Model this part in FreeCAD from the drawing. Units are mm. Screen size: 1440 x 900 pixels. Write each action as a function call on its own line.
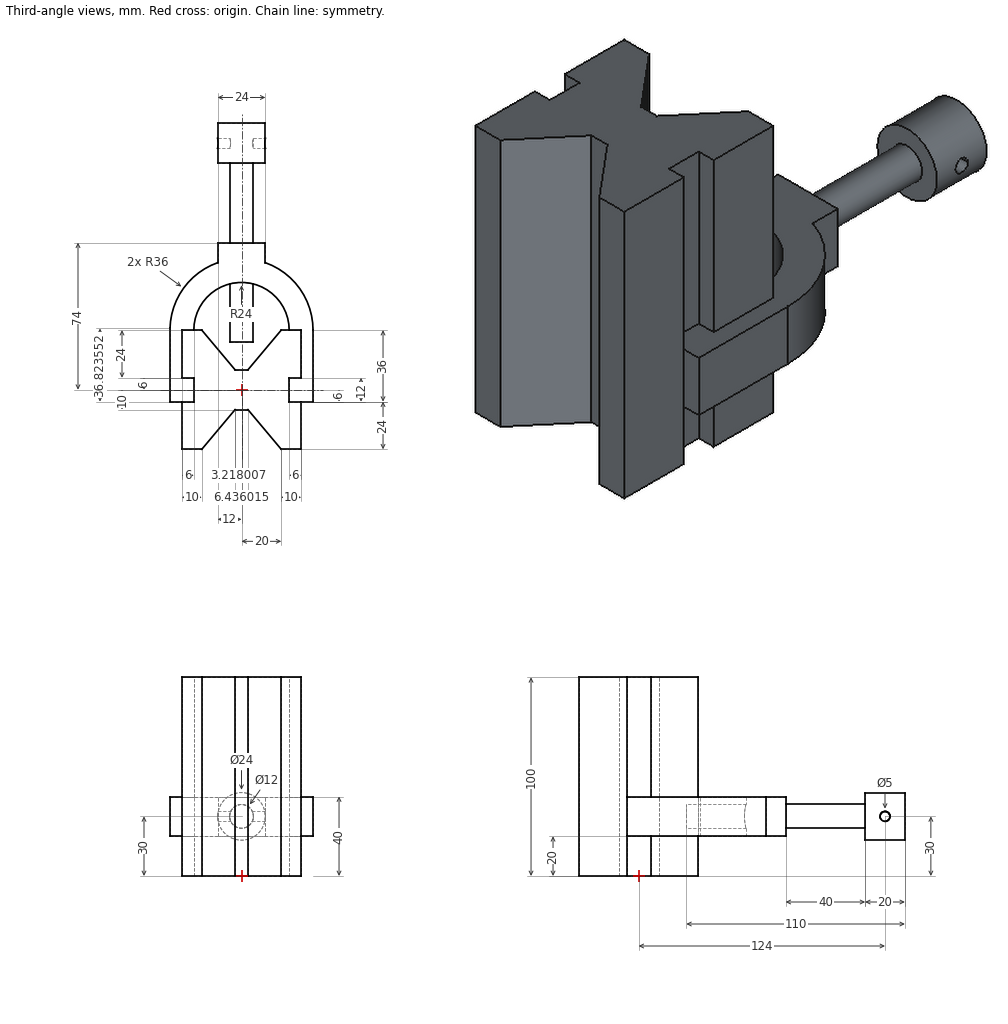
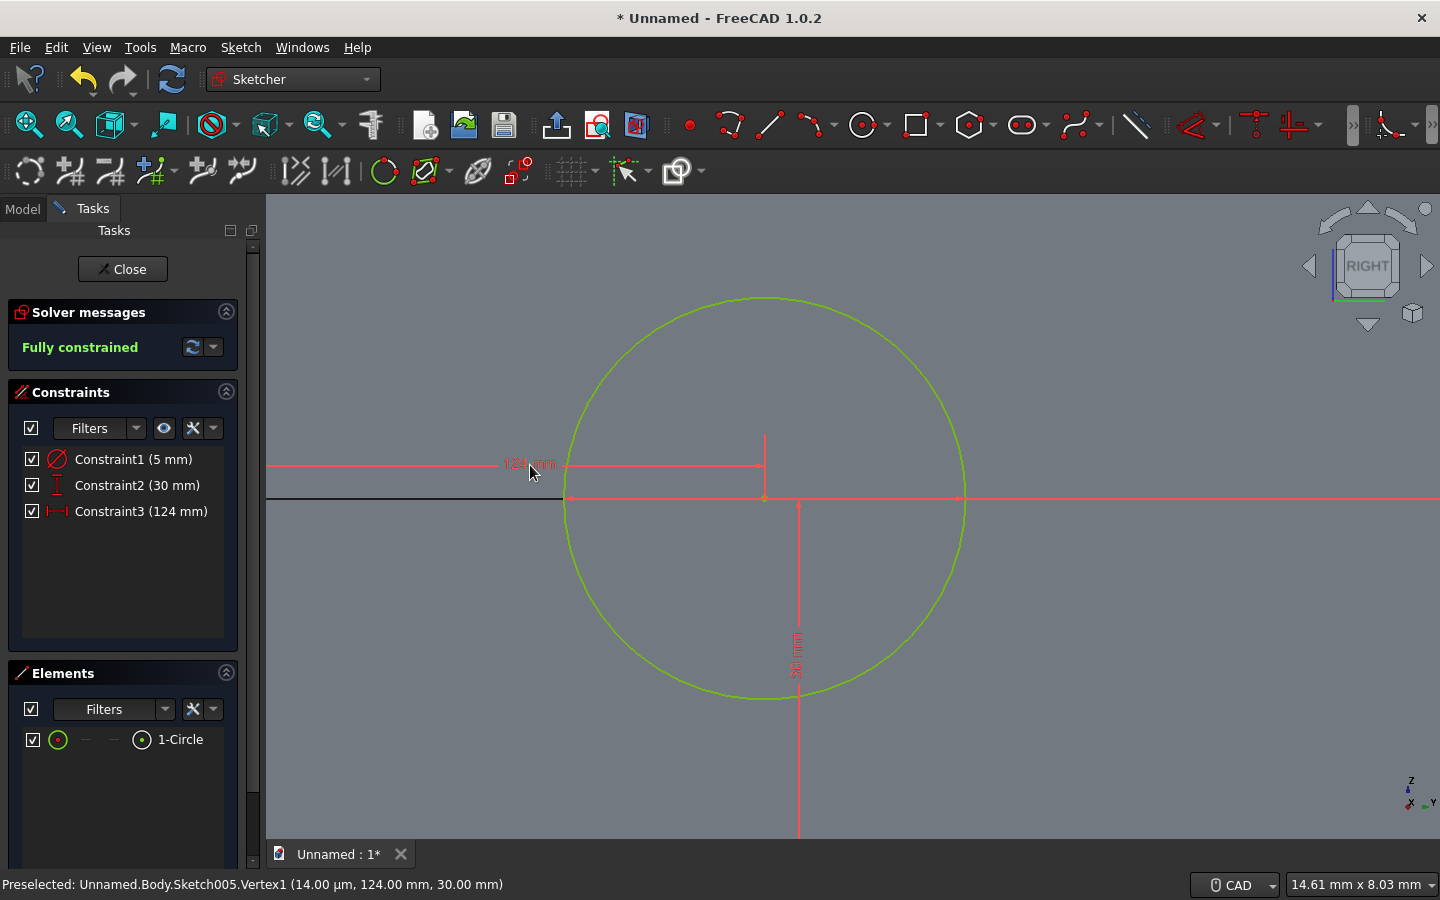
click(123, 269)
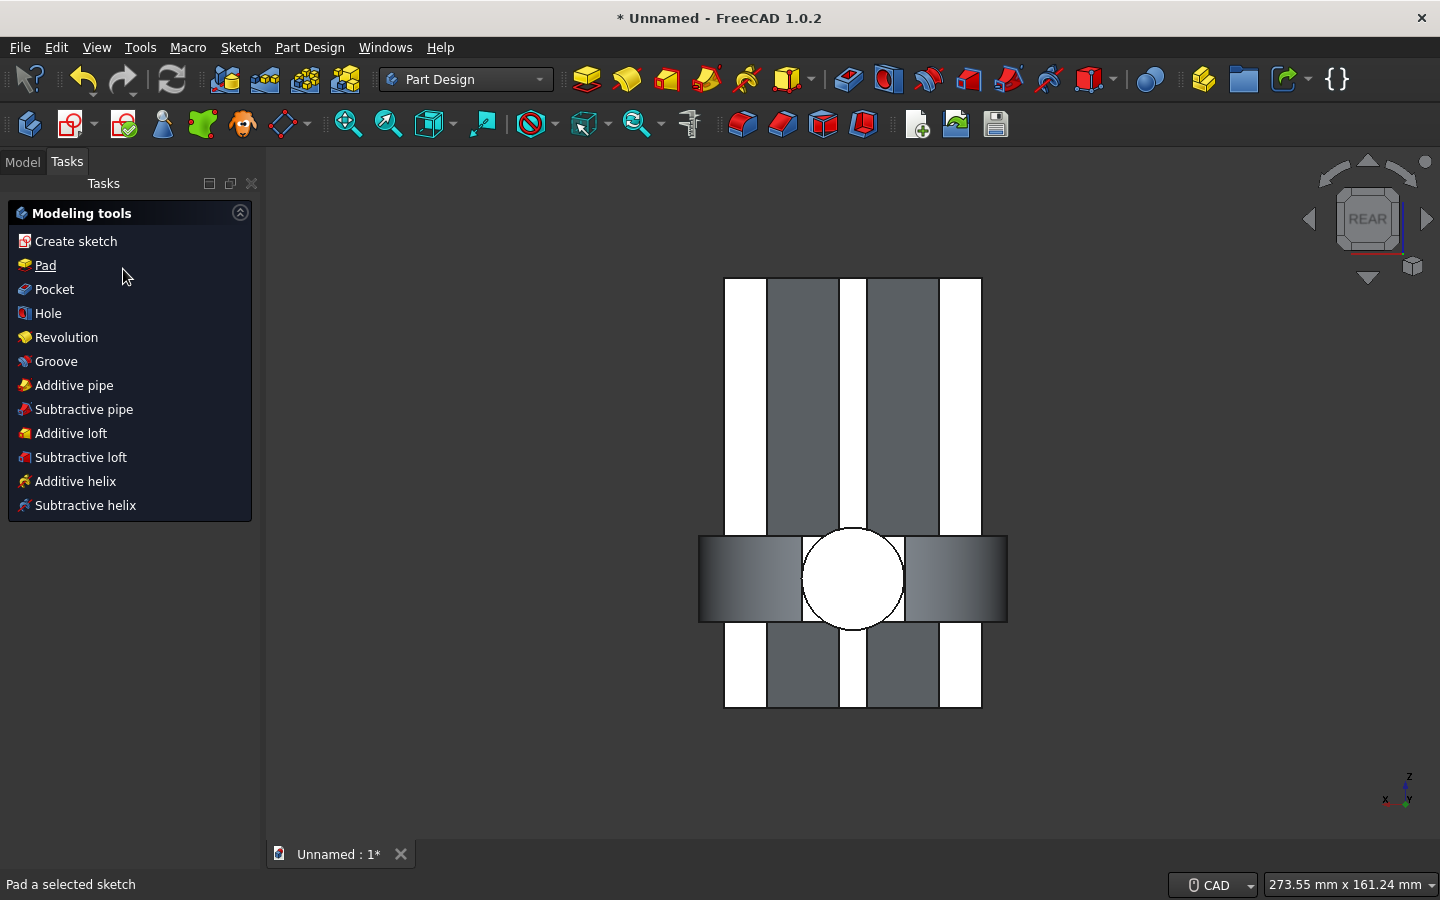
click(850, 80)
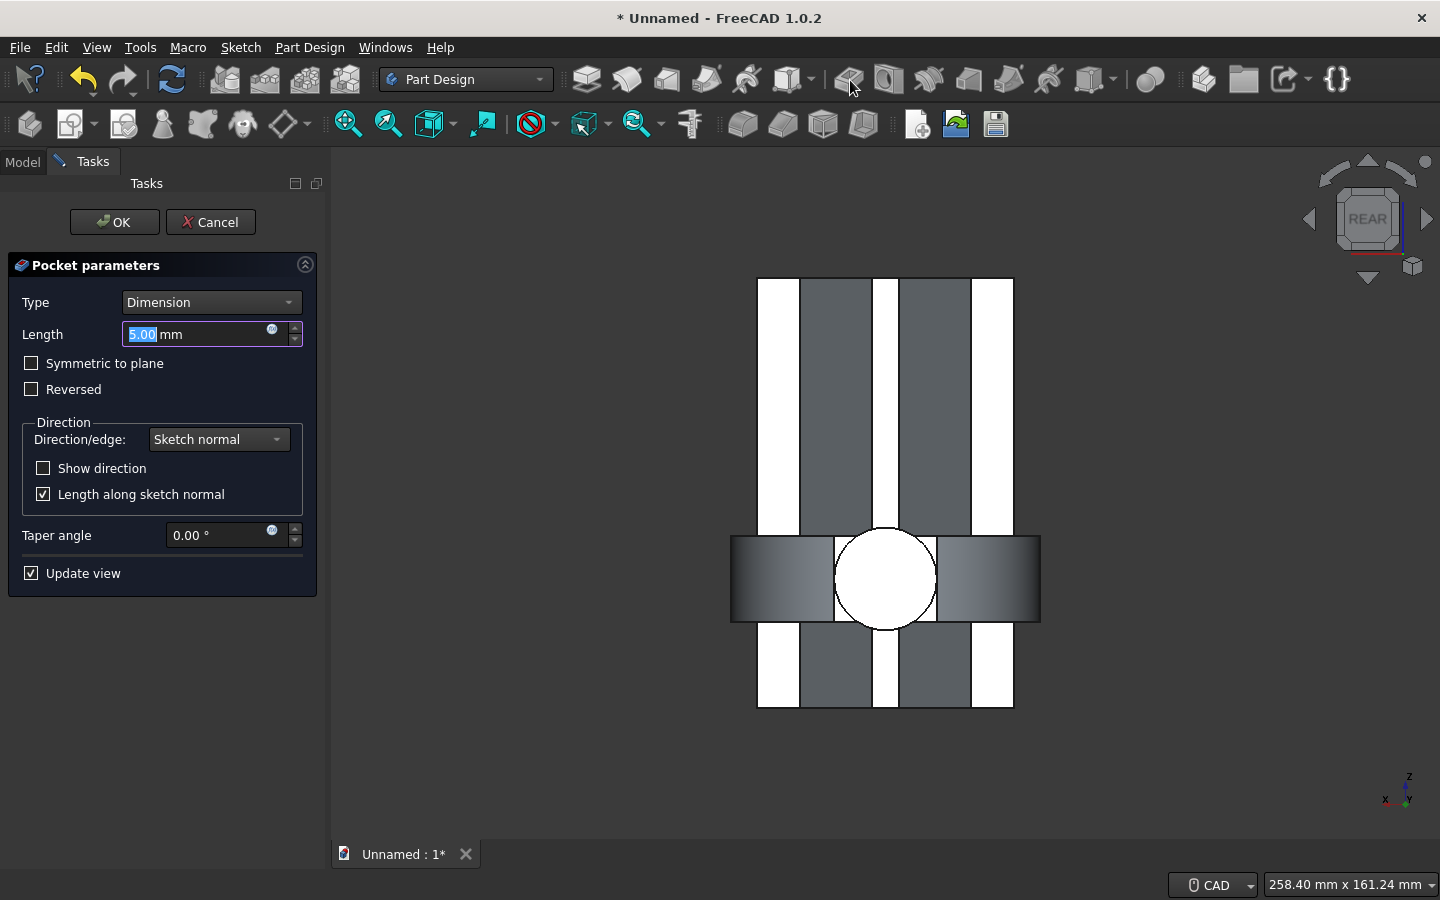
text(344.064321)
key(Tab)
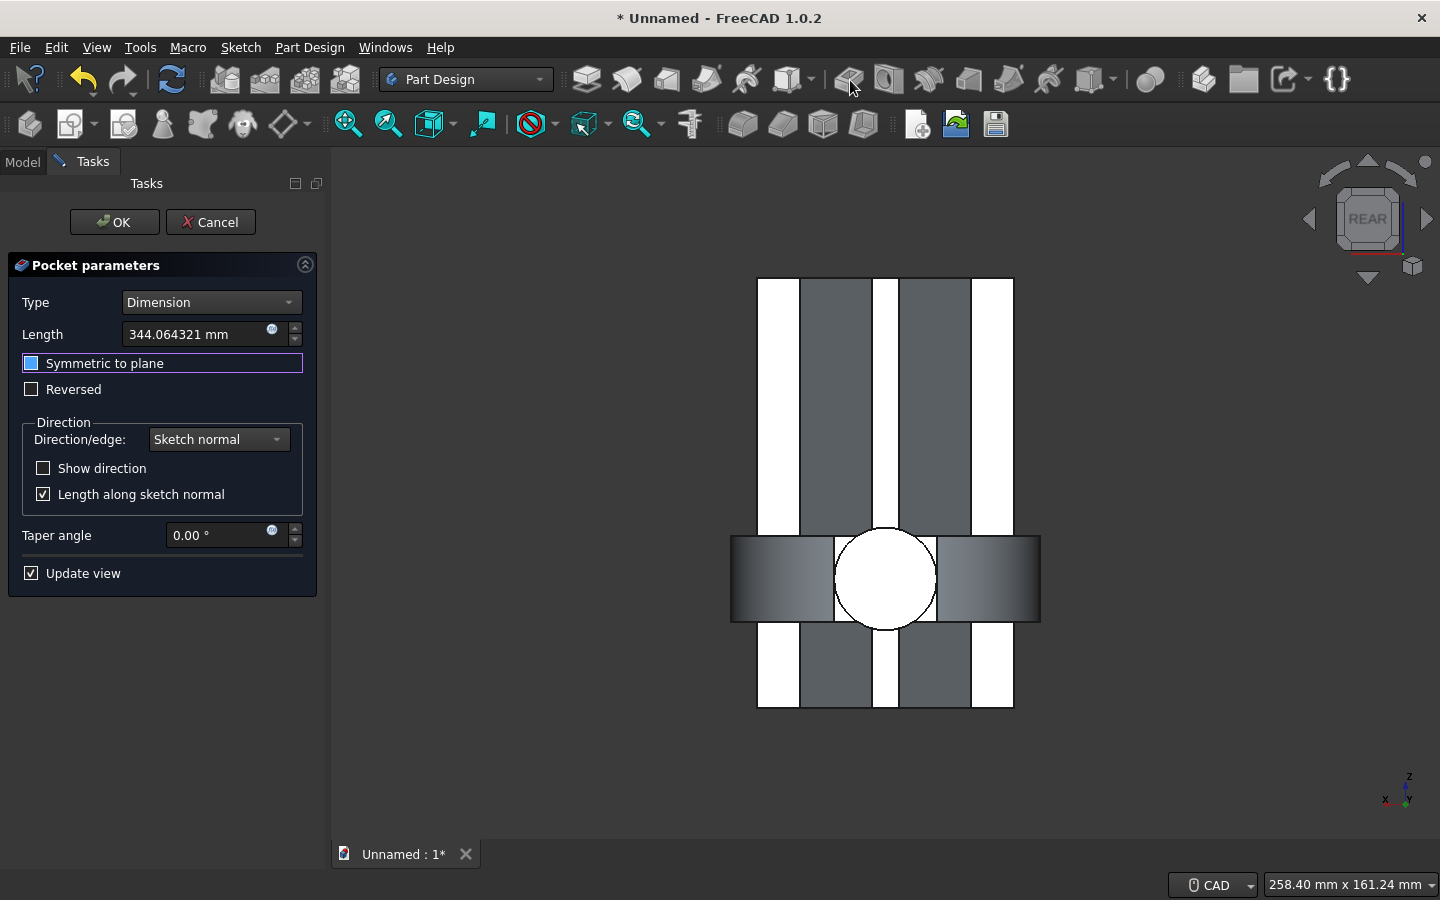
click(30, 363)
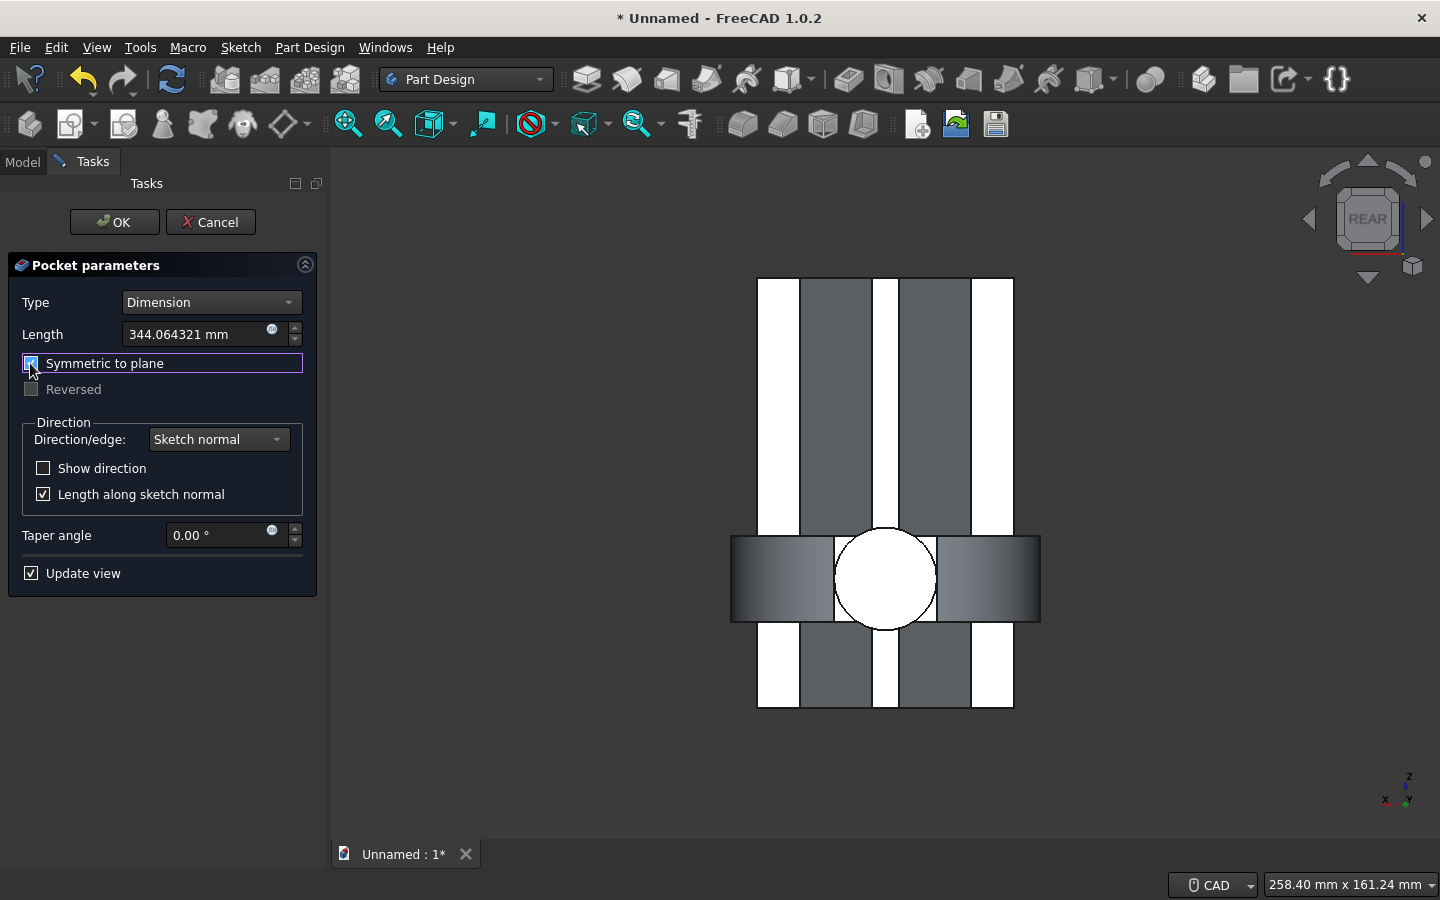
click(115, 222)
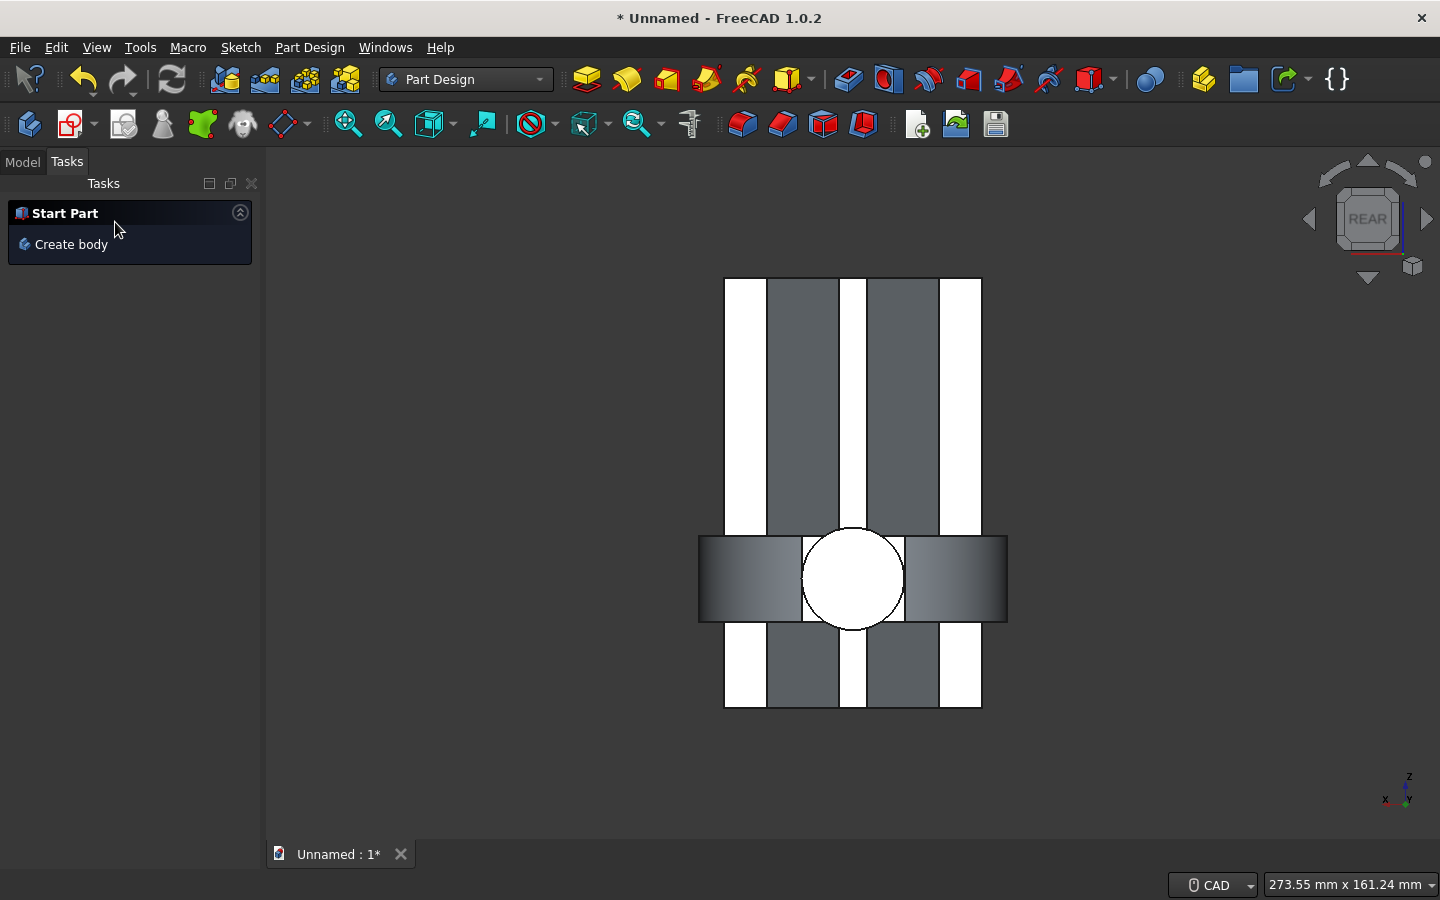
click(23, 161)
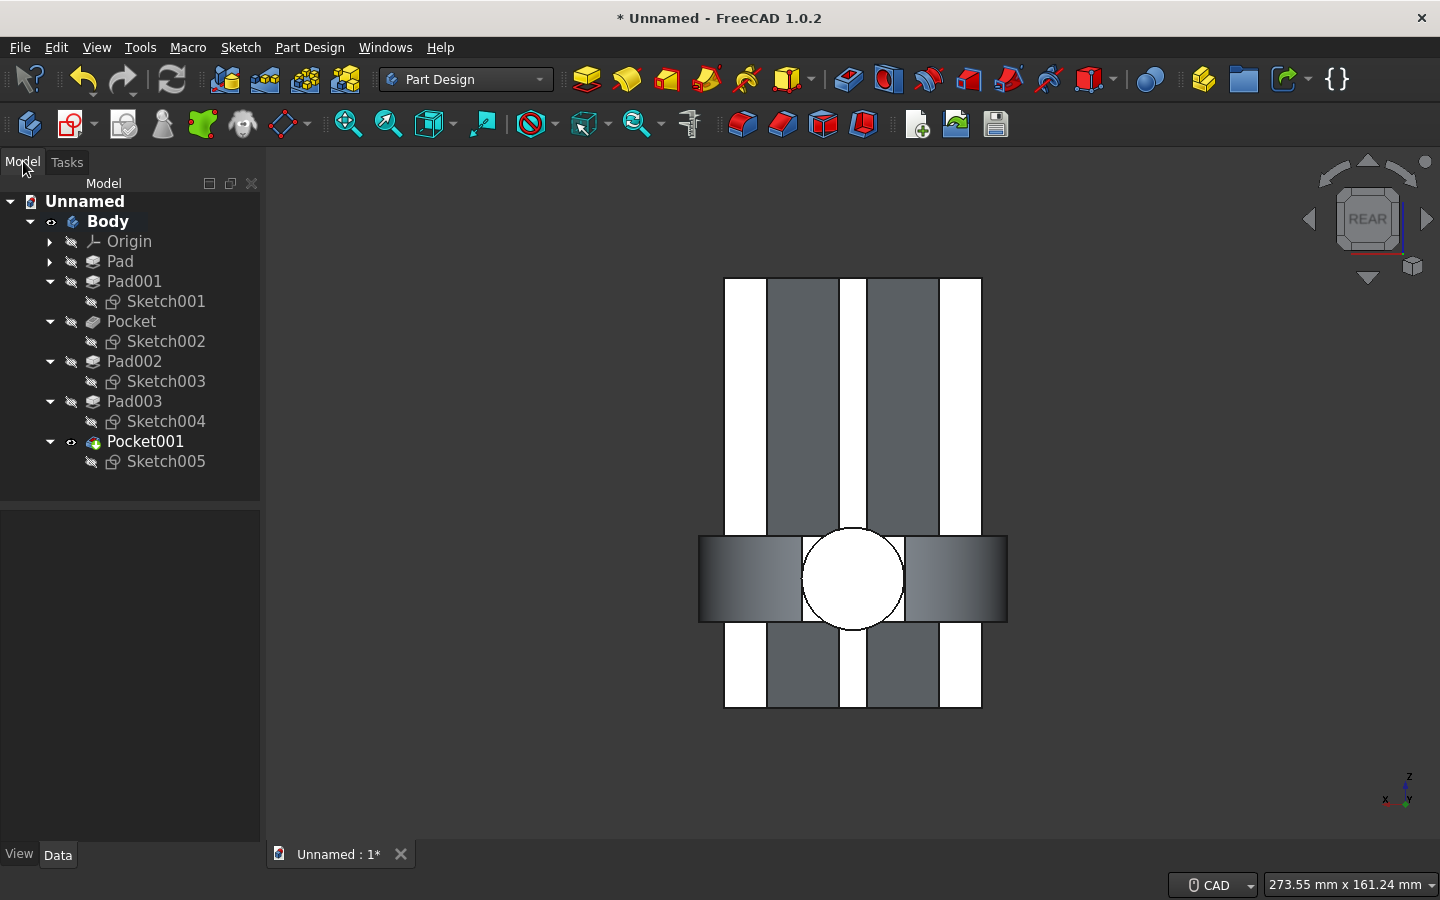
click(50, 242)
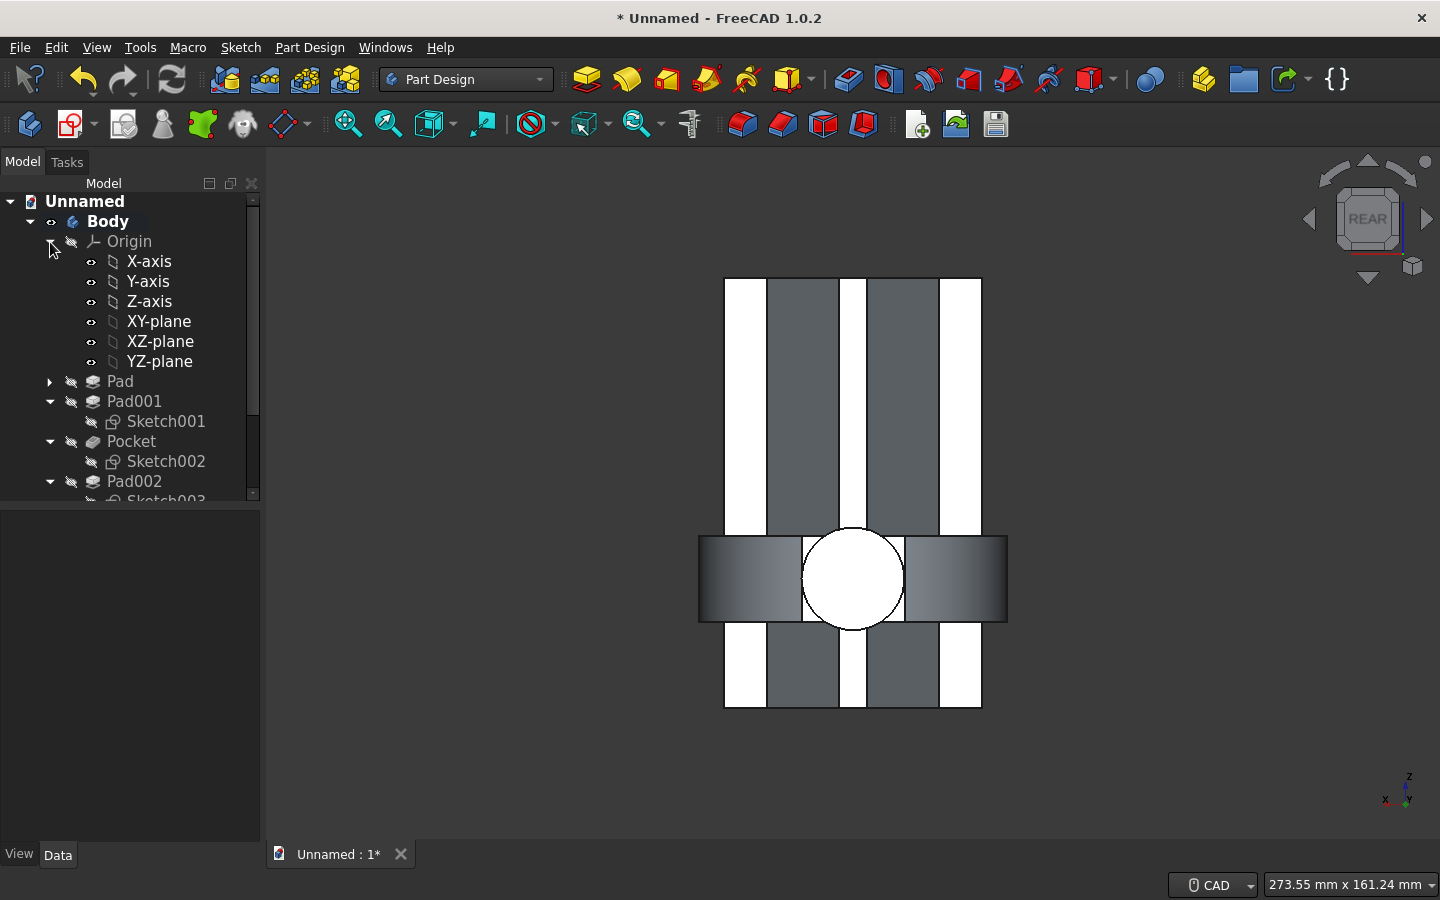
click(136, 342)